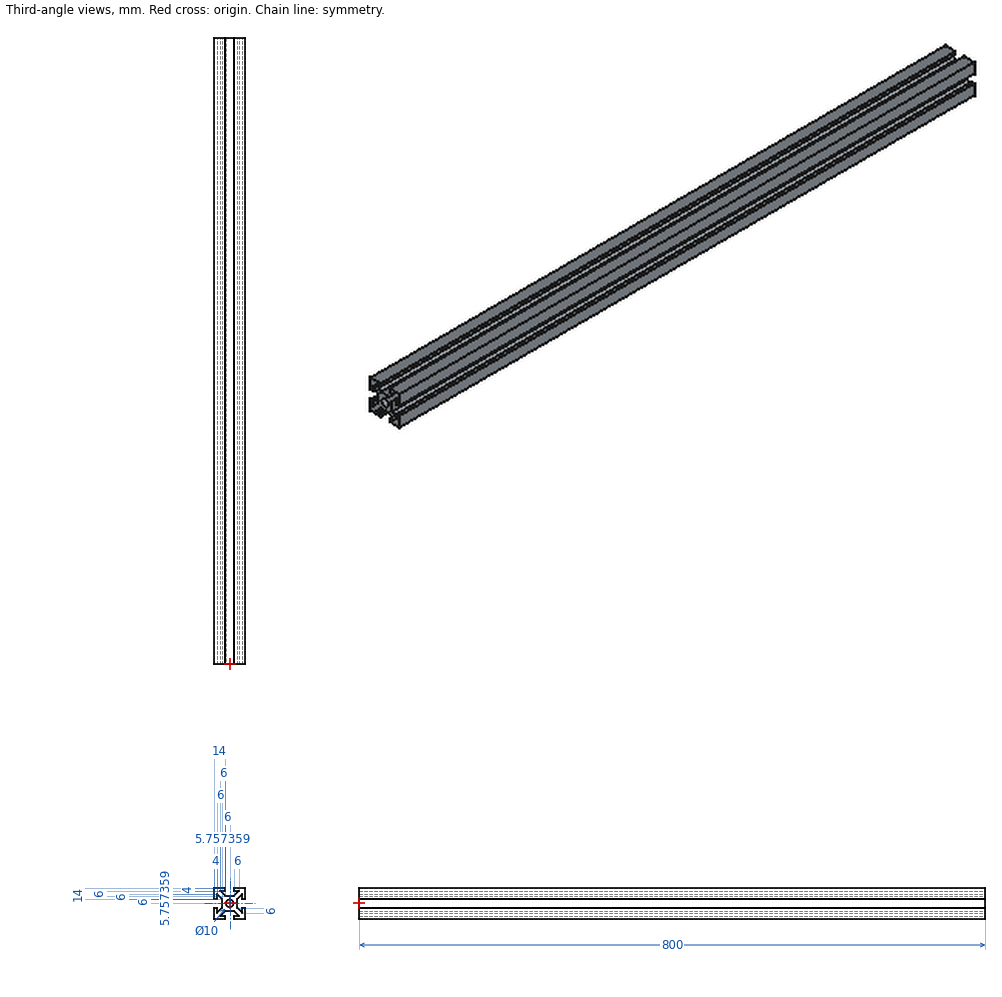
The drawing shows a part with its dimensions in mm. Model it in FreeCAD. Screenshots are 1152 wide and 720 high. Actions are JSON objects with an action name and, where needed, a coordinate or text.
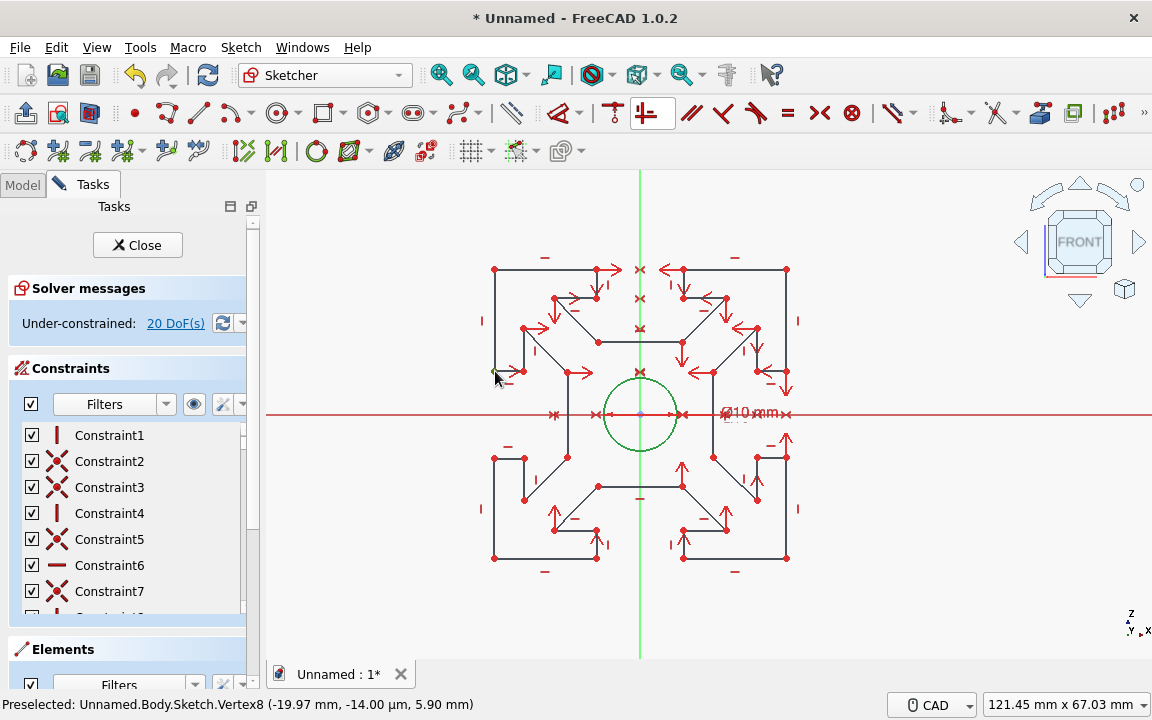
{"action": "left_click", "coordinate": [494, 459]}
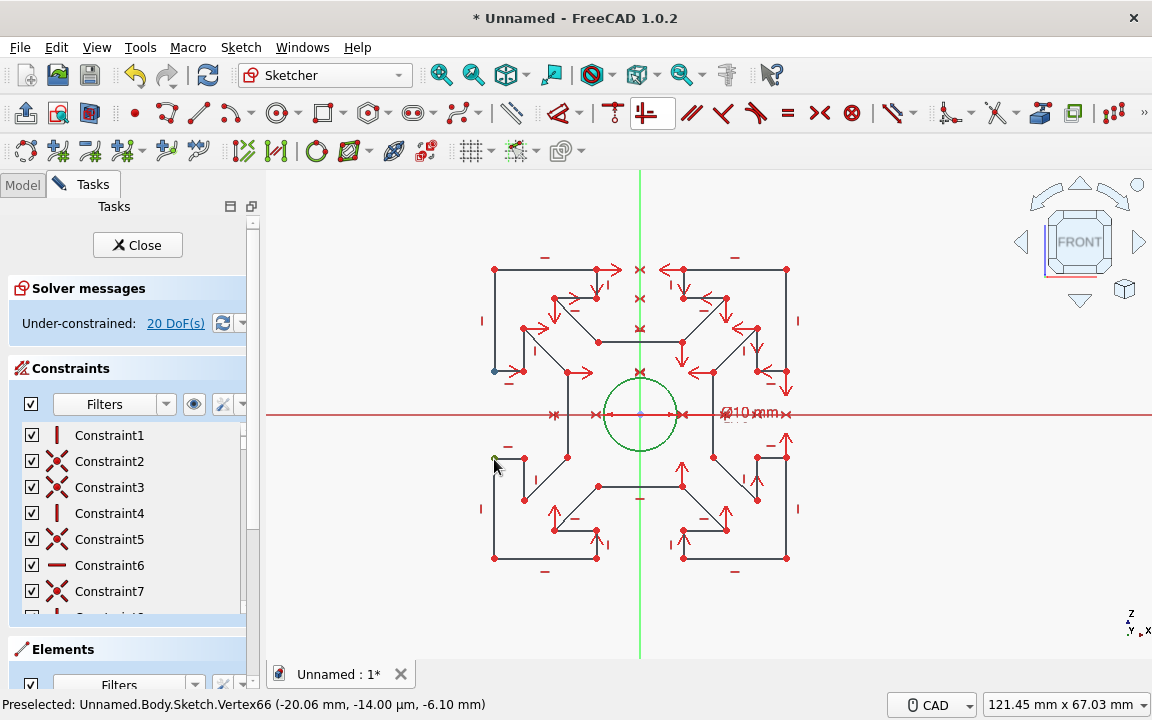
{"action": "left_click", "coordinate": [344, 414]}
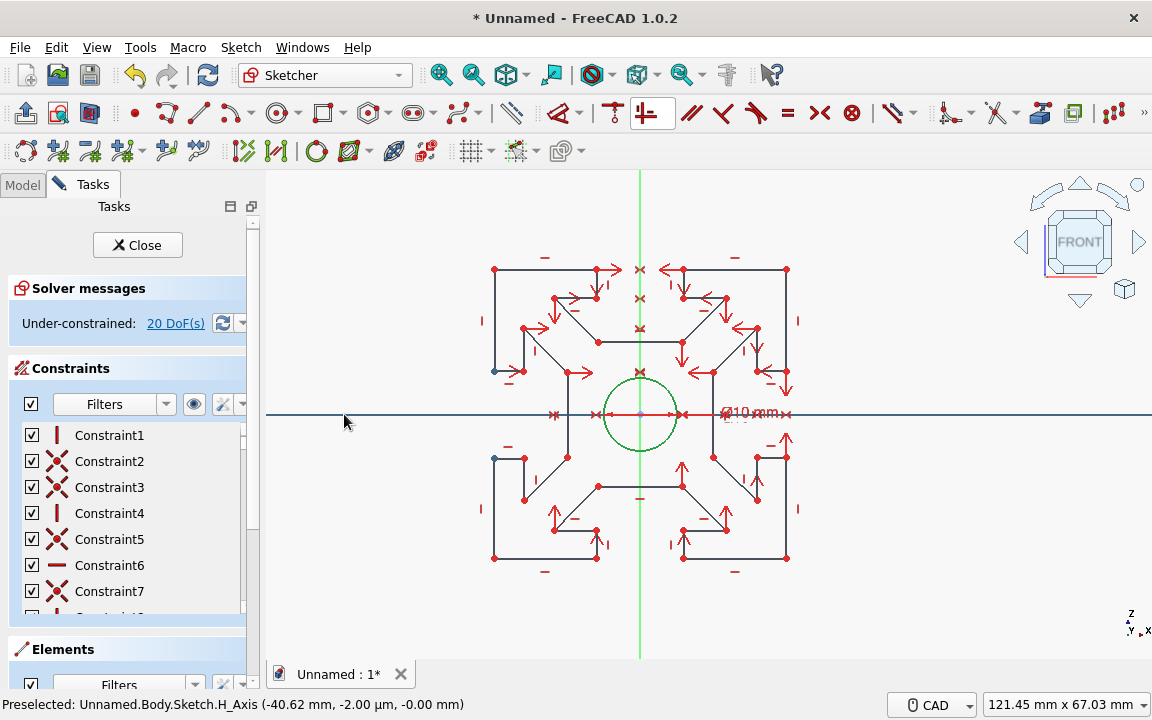
{"action": "key", "text": "s"}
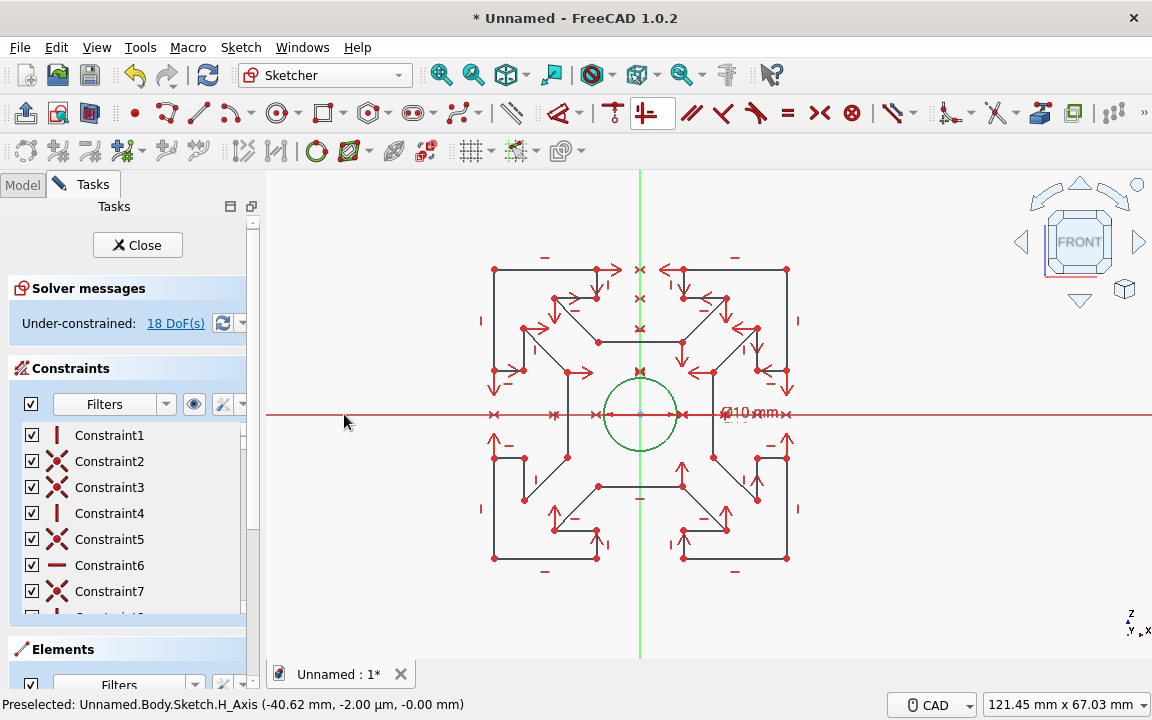
{"action": "left_click", "coordinate": [524, 329]}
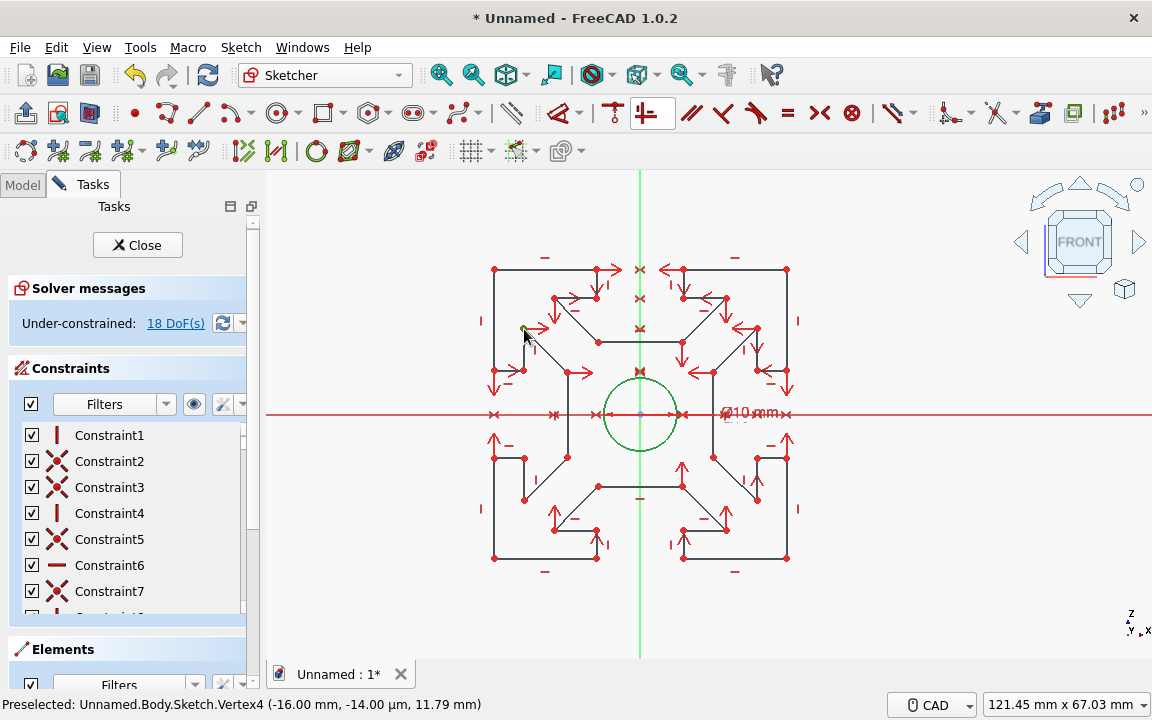
{"action": "left_click", "coordinate": [524, 501]}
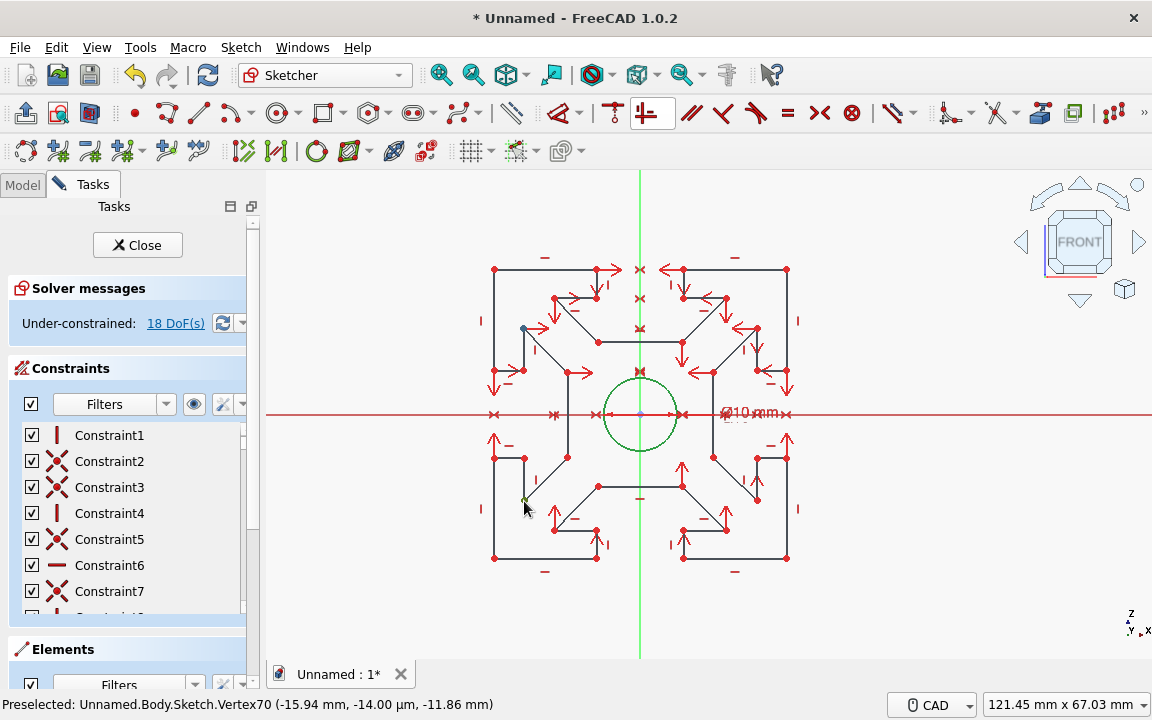
{"action": "left_click", "coordinate": [344, 414]}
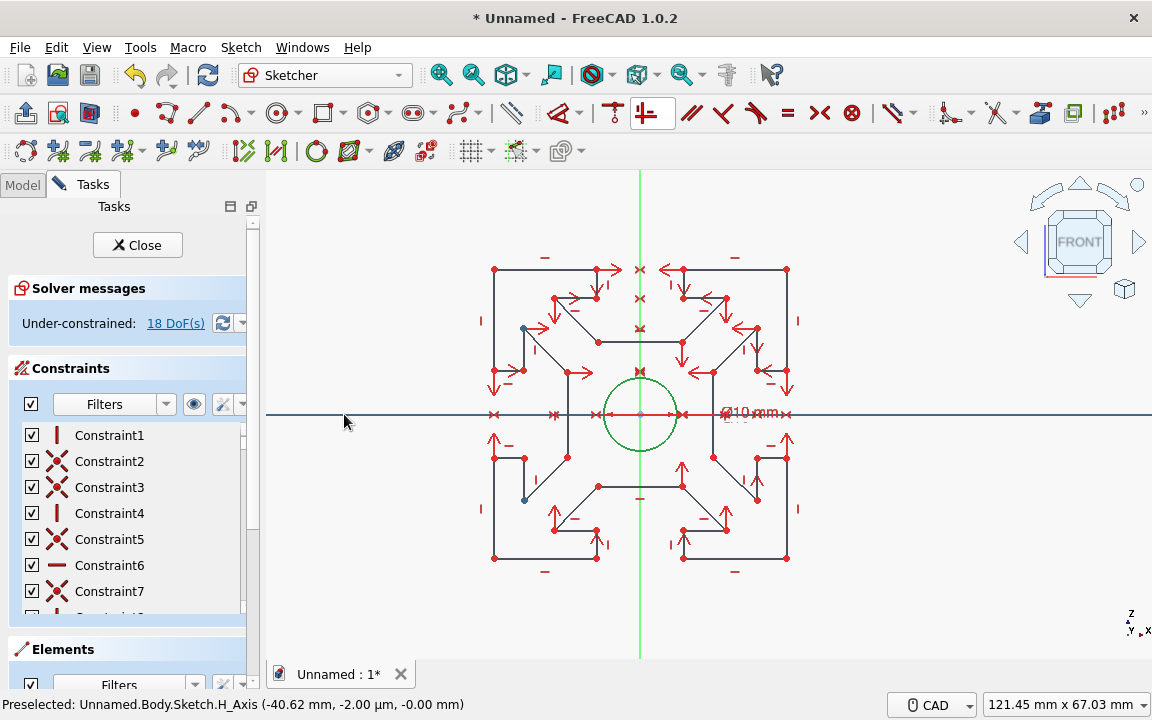
{"action": "key", "text": "s"}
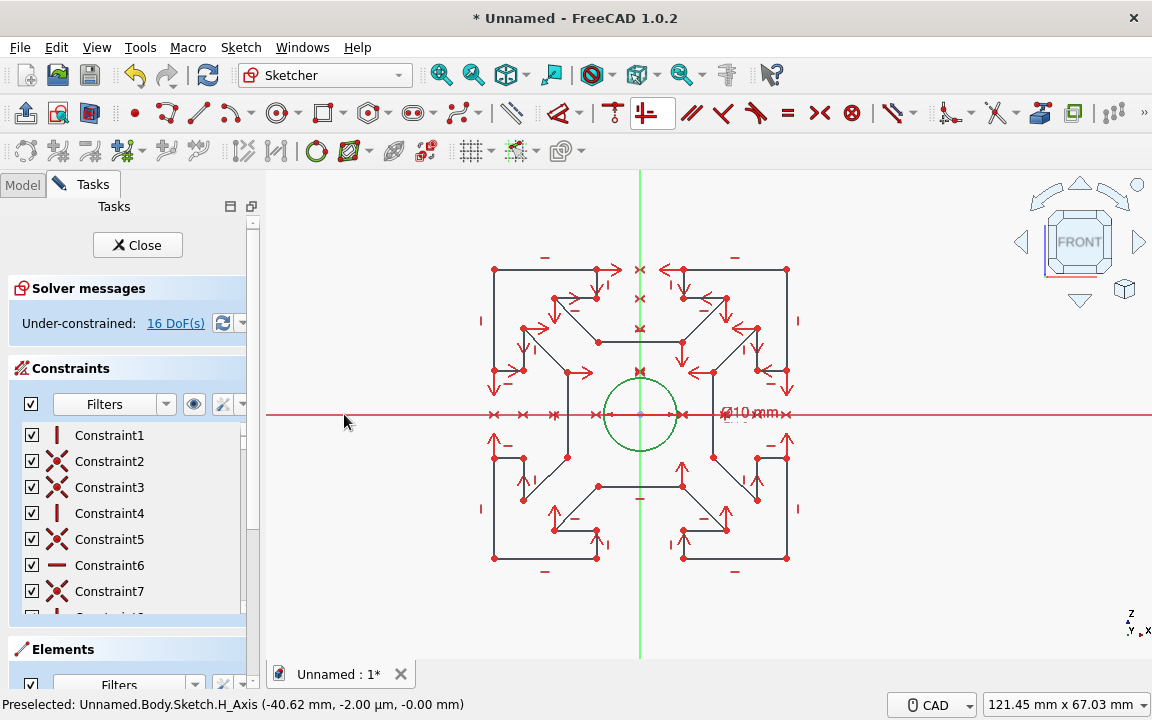
{"action": "key", "text": "d"}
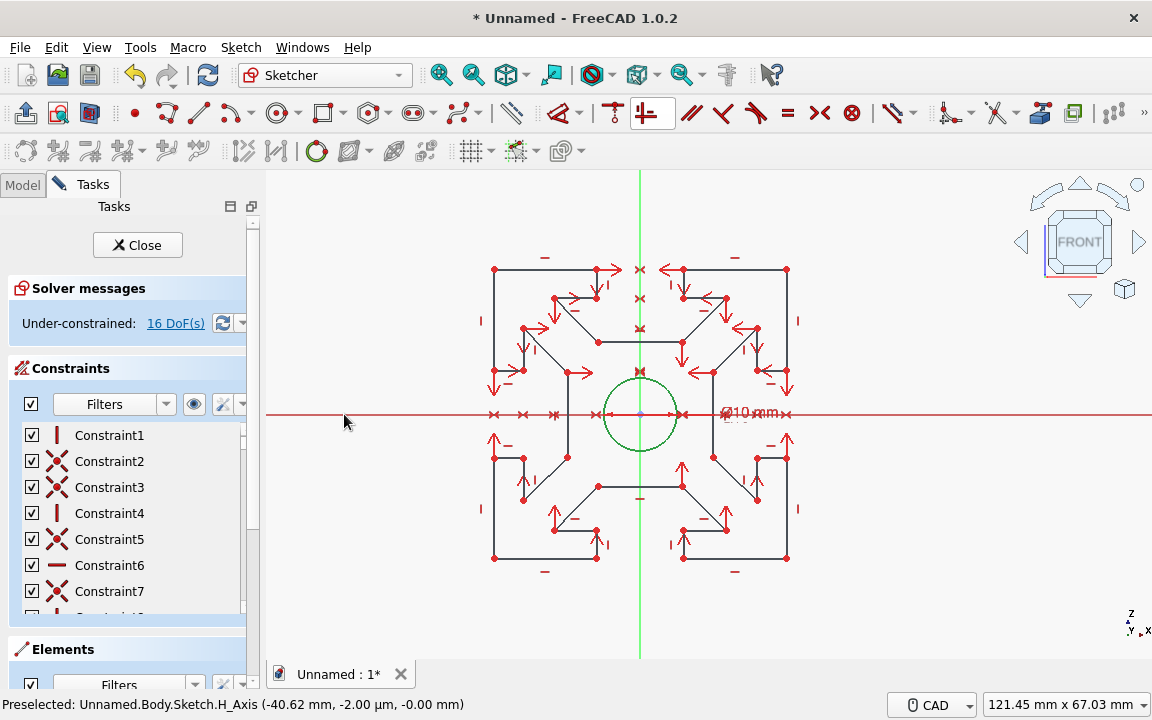
{"action": "scroll", "coordinate": [512, 371], "scroll_direction": "up", "scroll_amount": 2}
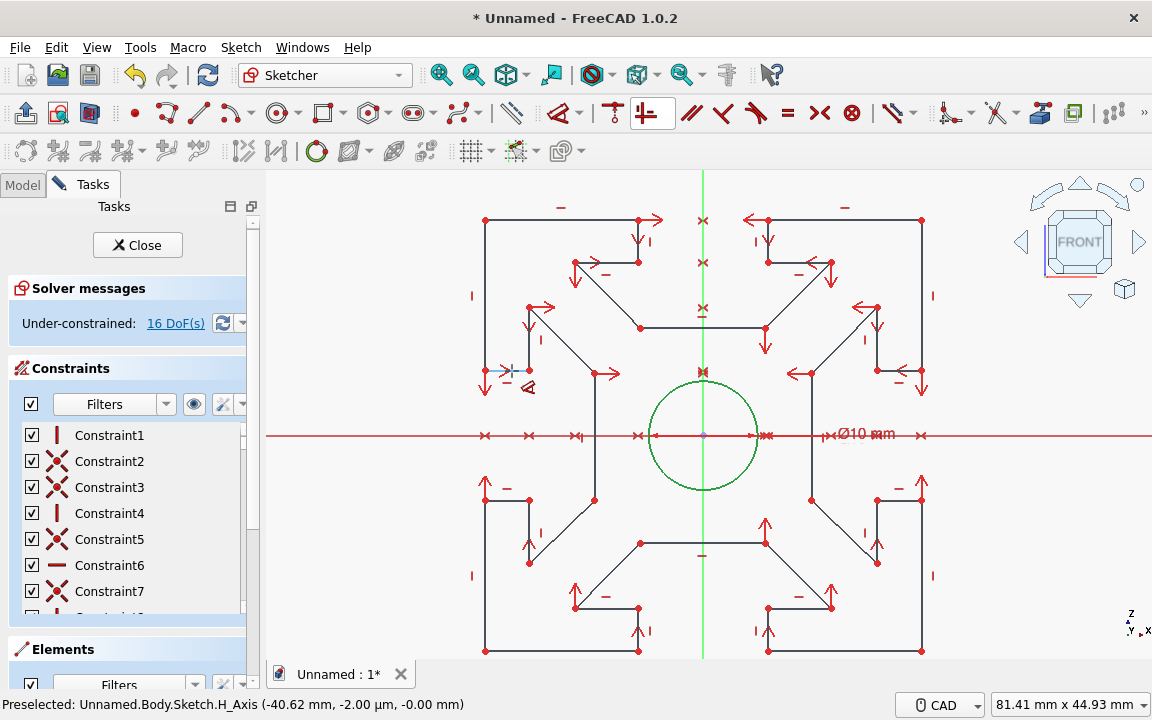
{"action": "left_click", "coordinate": [512, 371]}
{"action": "left_click", "coordinate": [507, 337]}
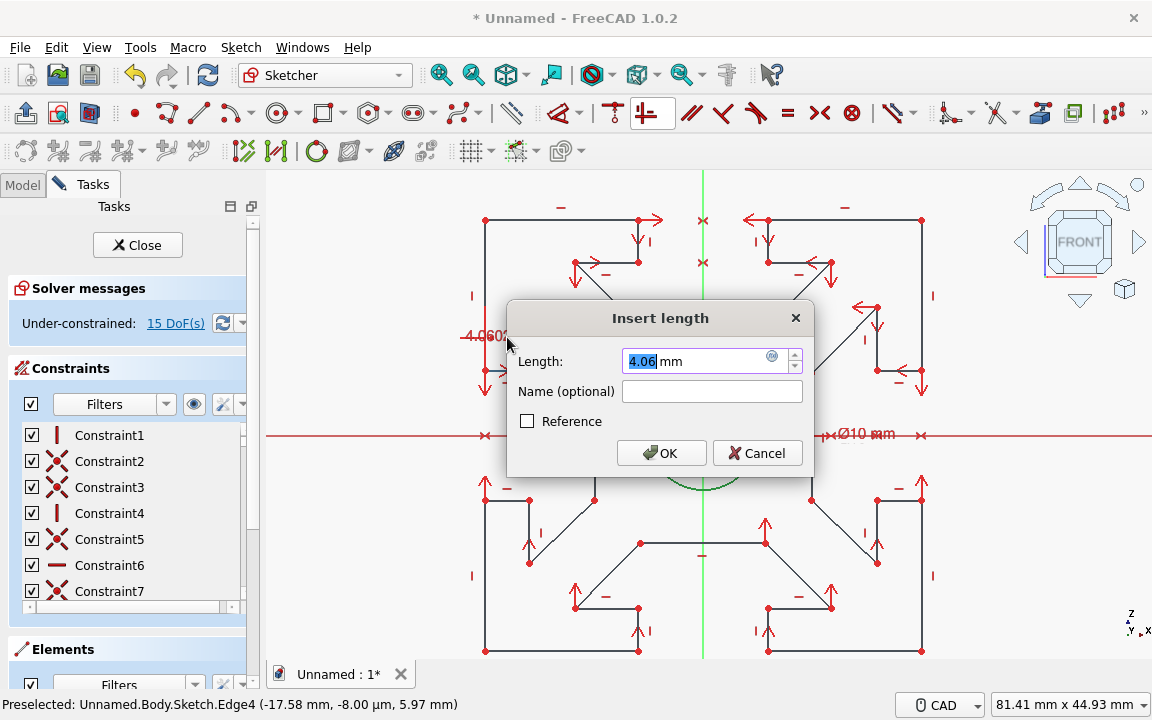
{"action": "type", "text": "4"}
{"action": "key", "text": "Return"}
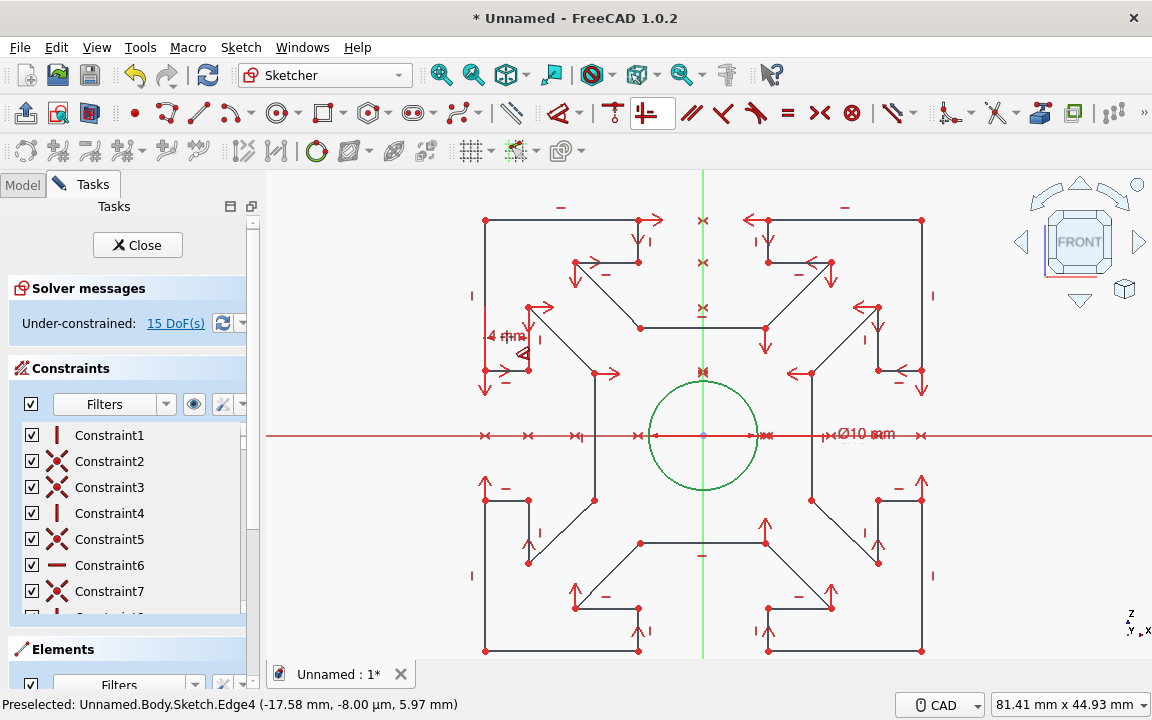
{"action": "left_click", "coordinate": [638, 233]}
{"action": "left_click", "coordinate": [604, 241]}